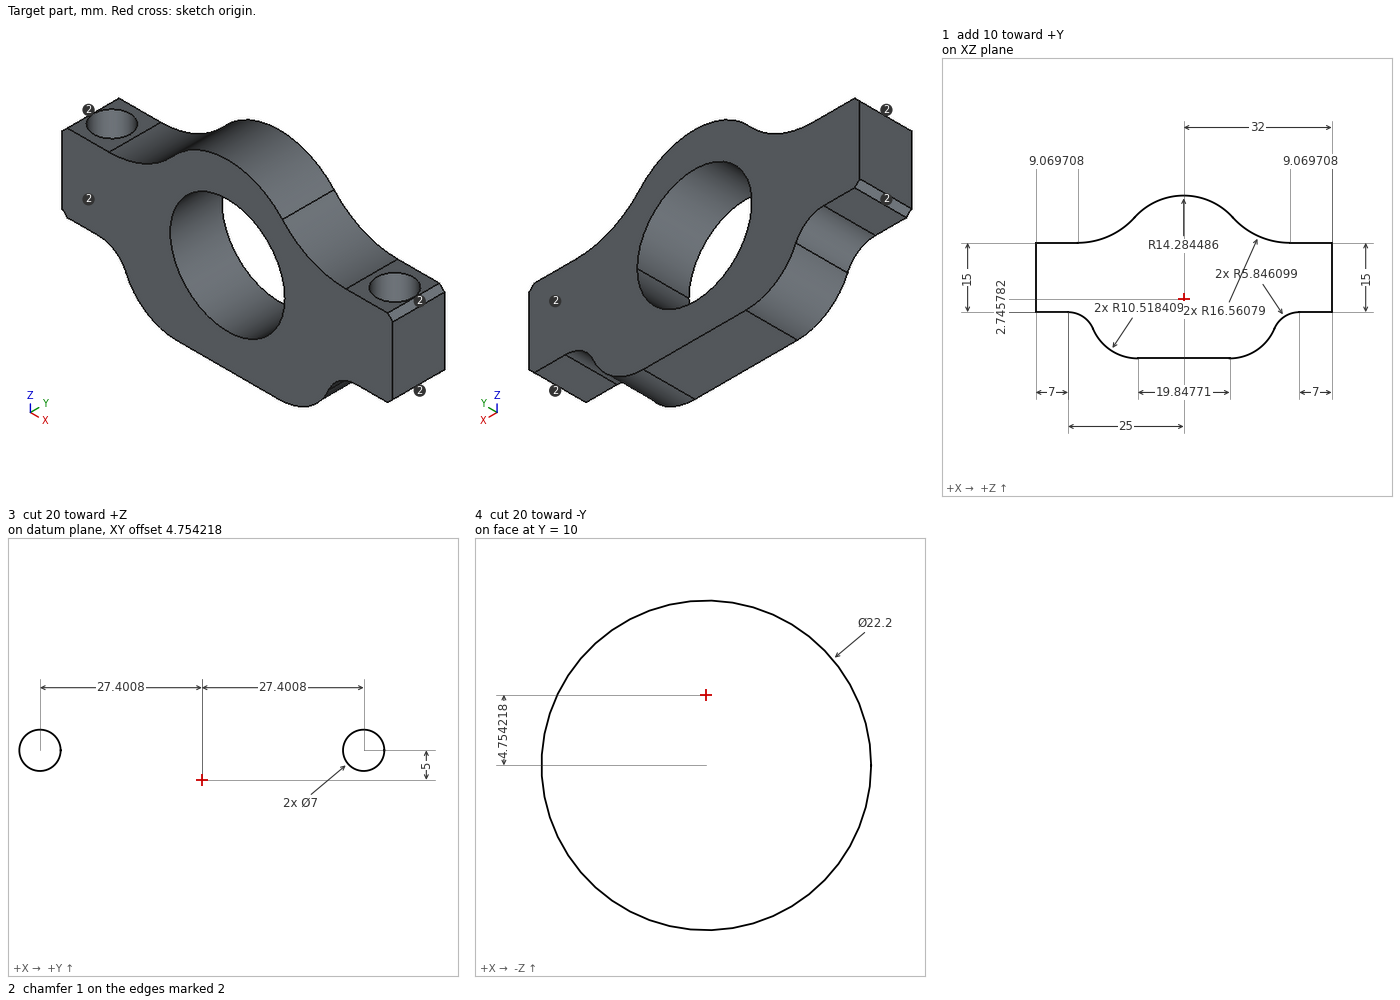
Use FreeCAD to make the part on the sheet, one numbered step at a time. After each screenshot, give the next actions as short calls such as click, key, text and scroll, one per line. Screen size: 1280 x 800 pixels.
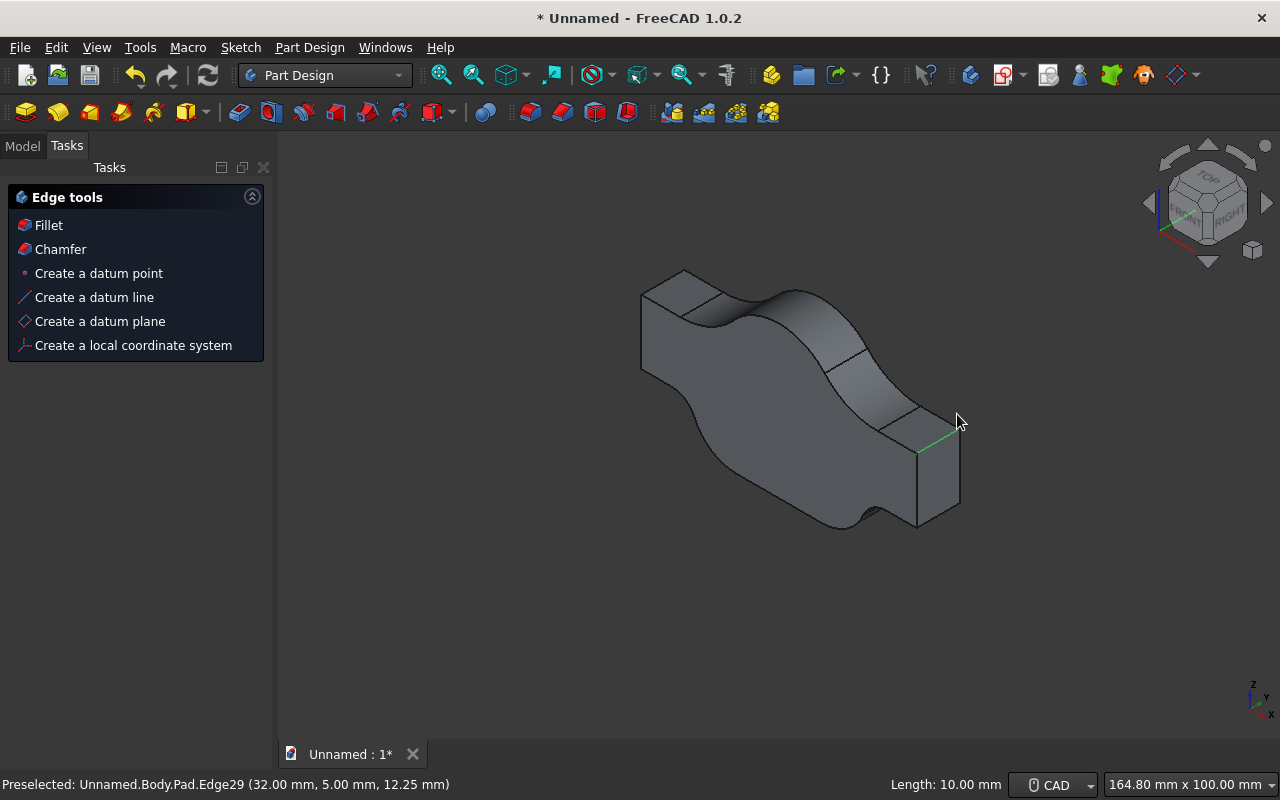
key(2)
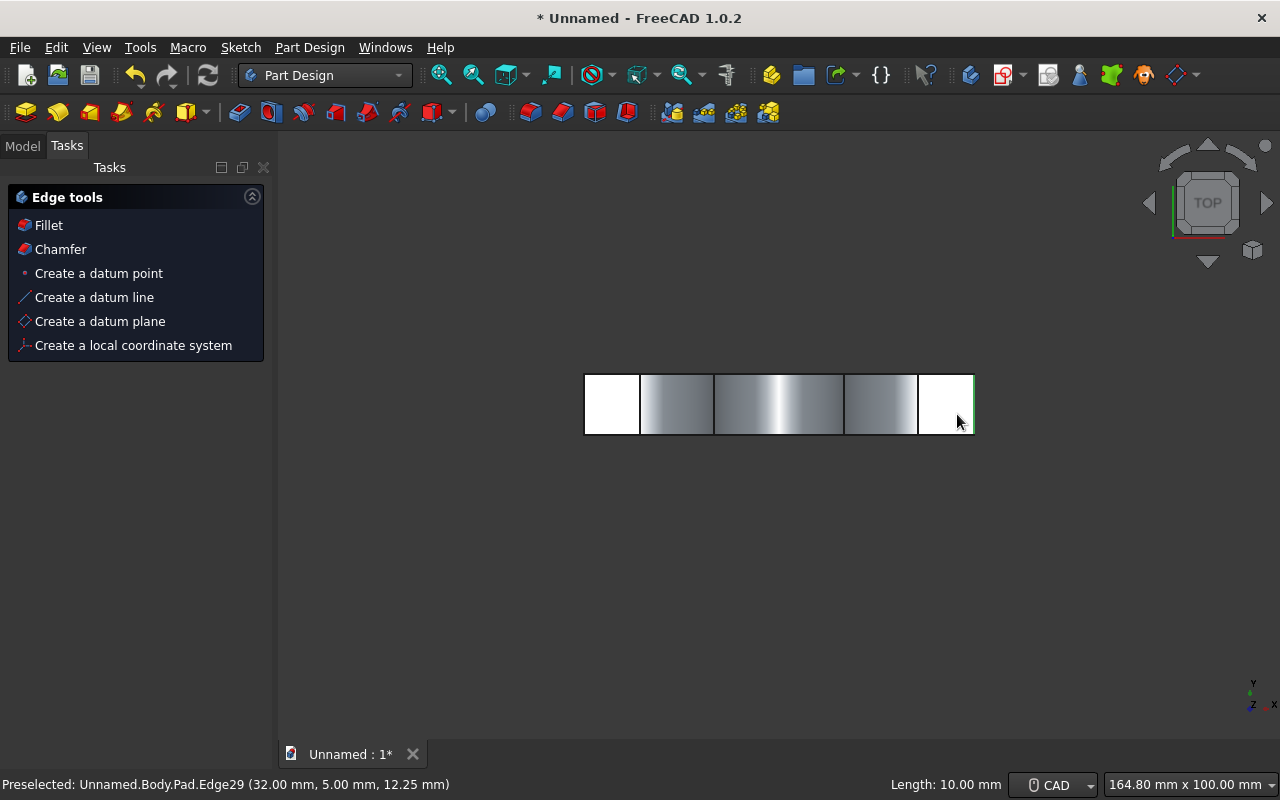
click(442, 76)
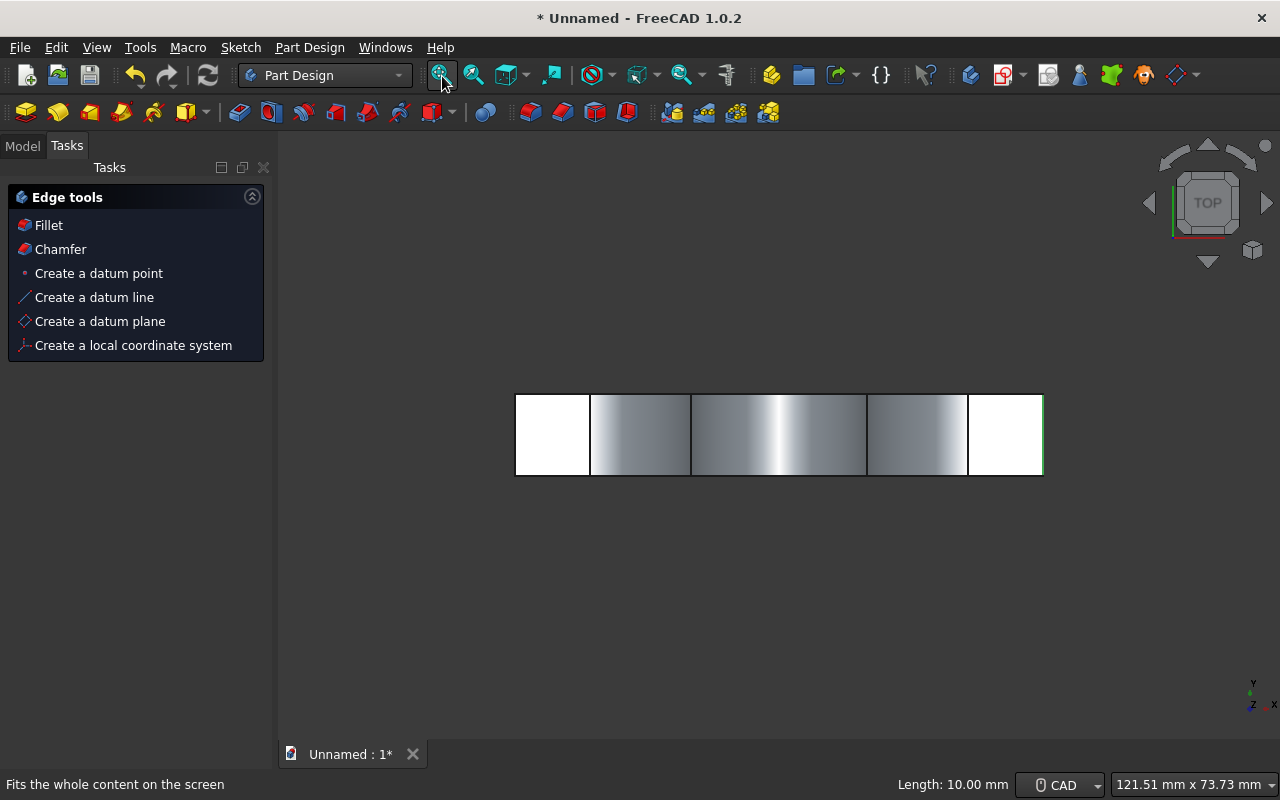
click(515, 434, ctrl)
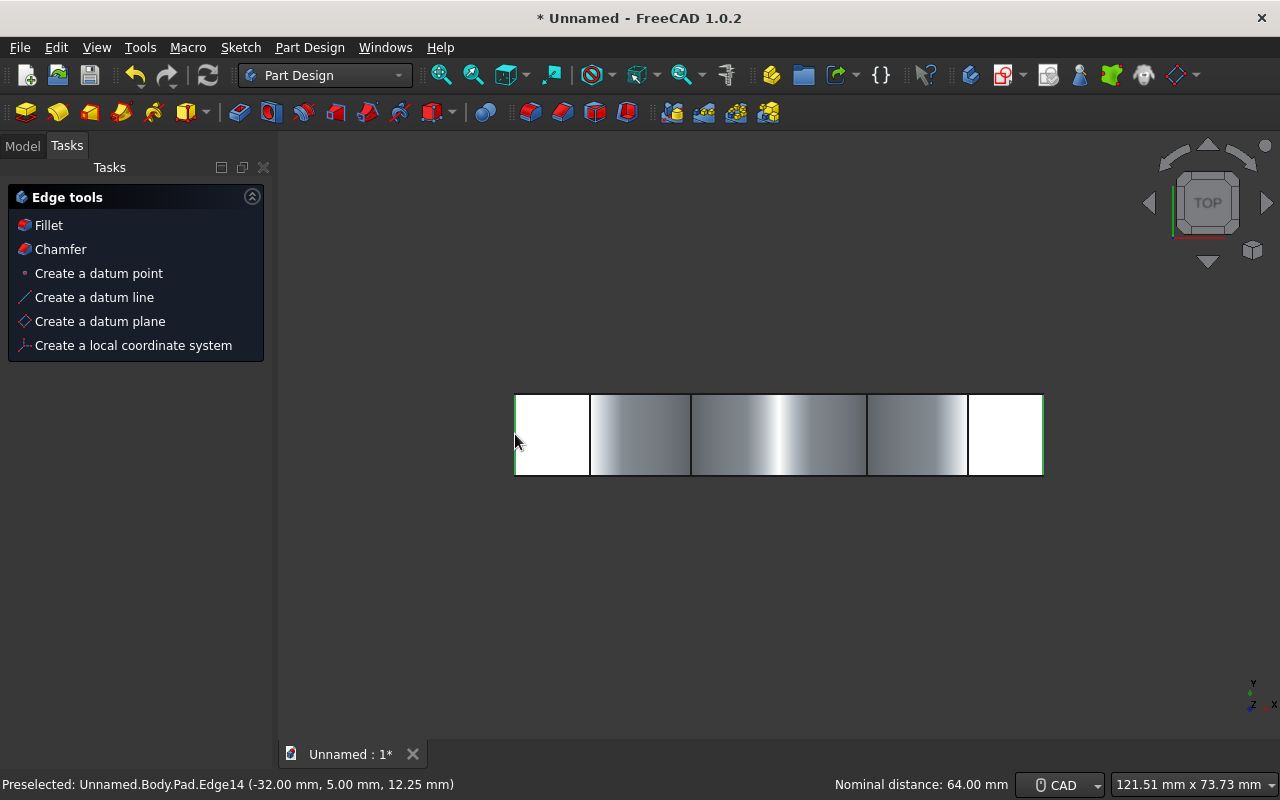
key(1)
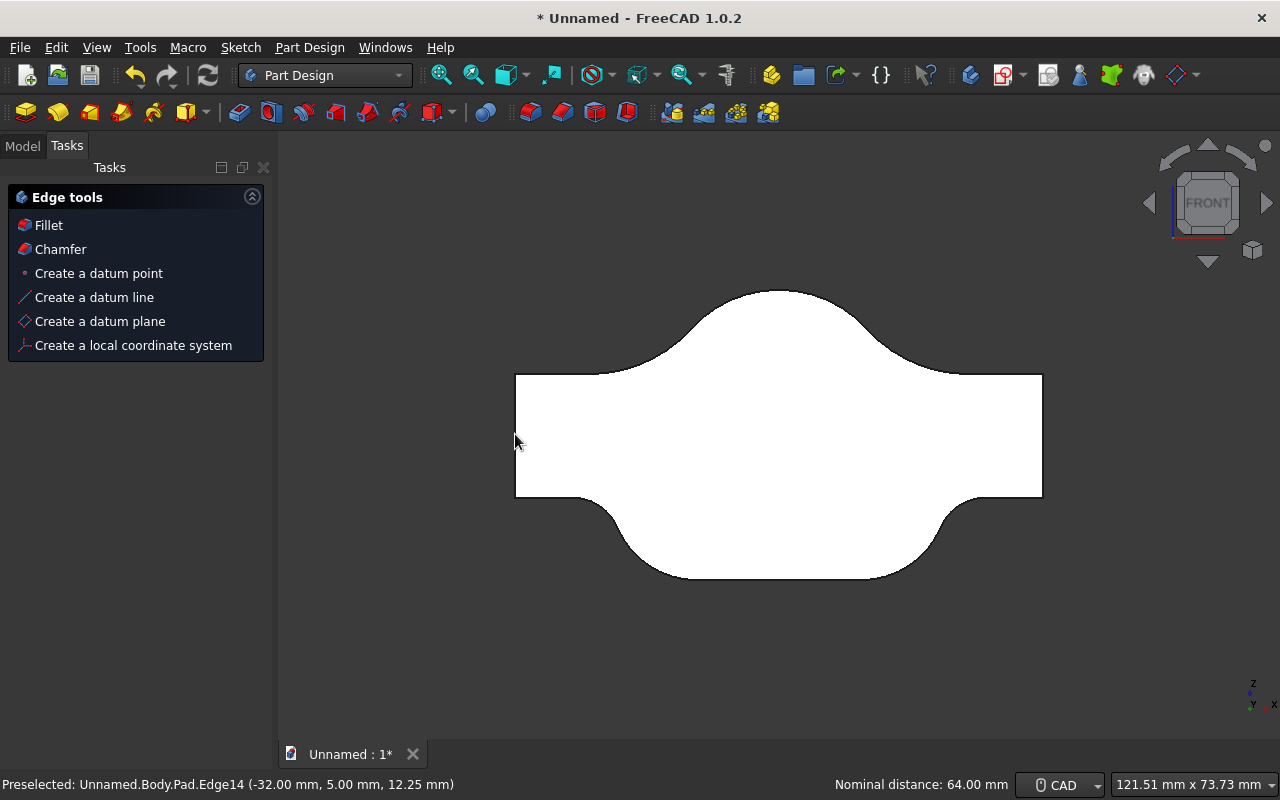
key(3)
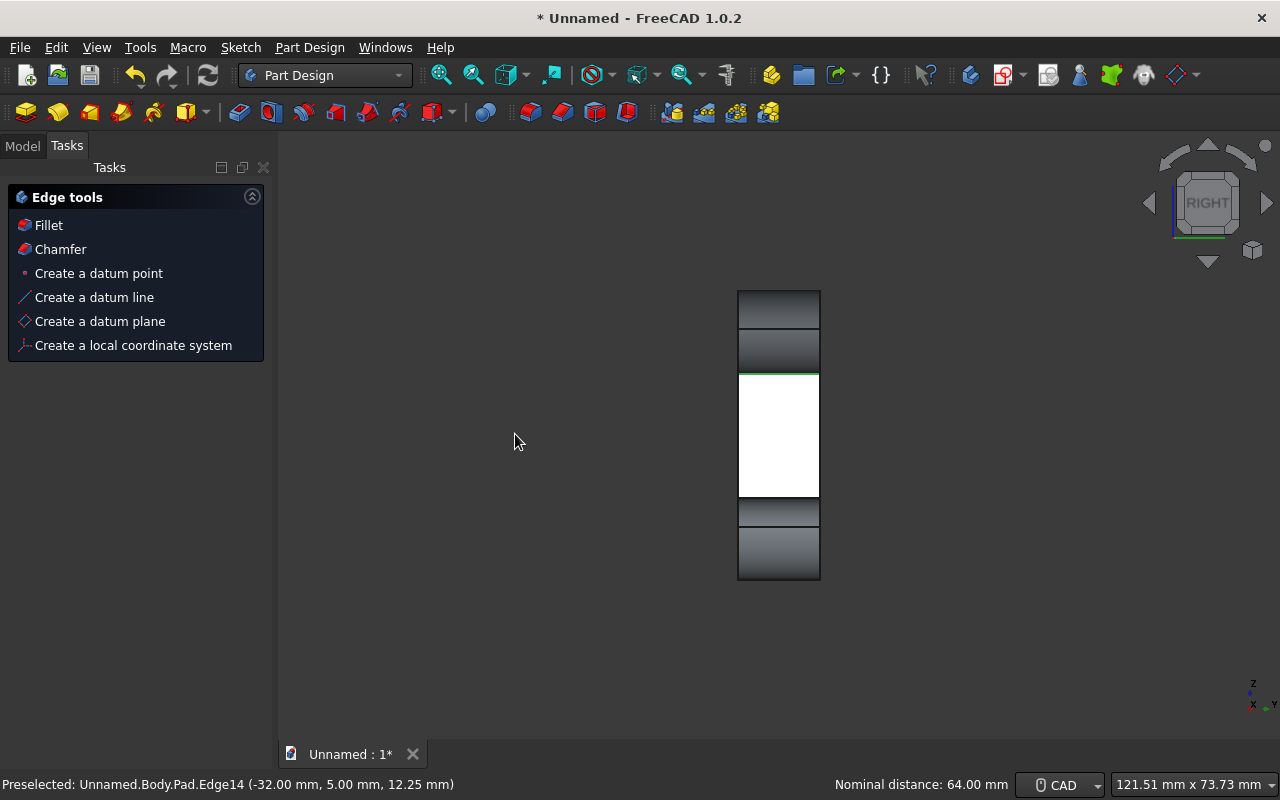
click(779, 497, ctrl)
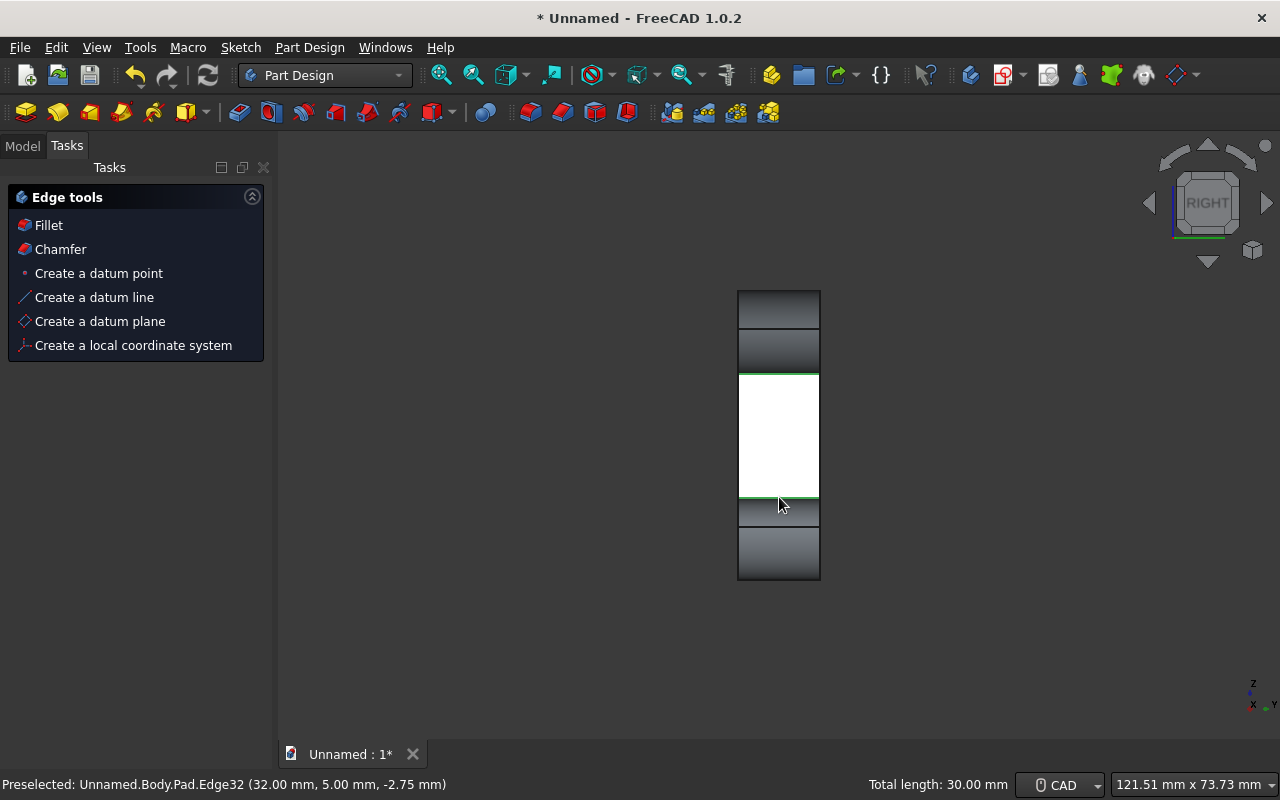
key(5)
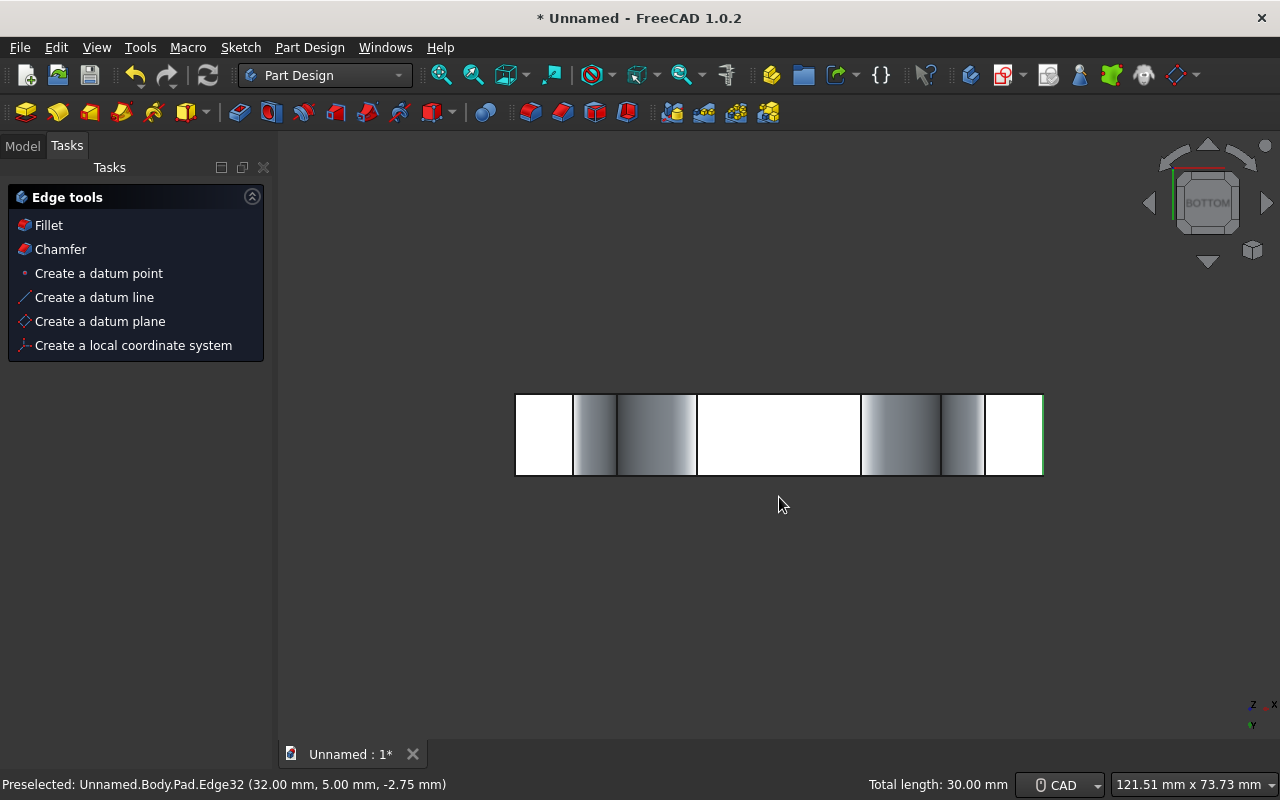
click(515, 434, ctrl)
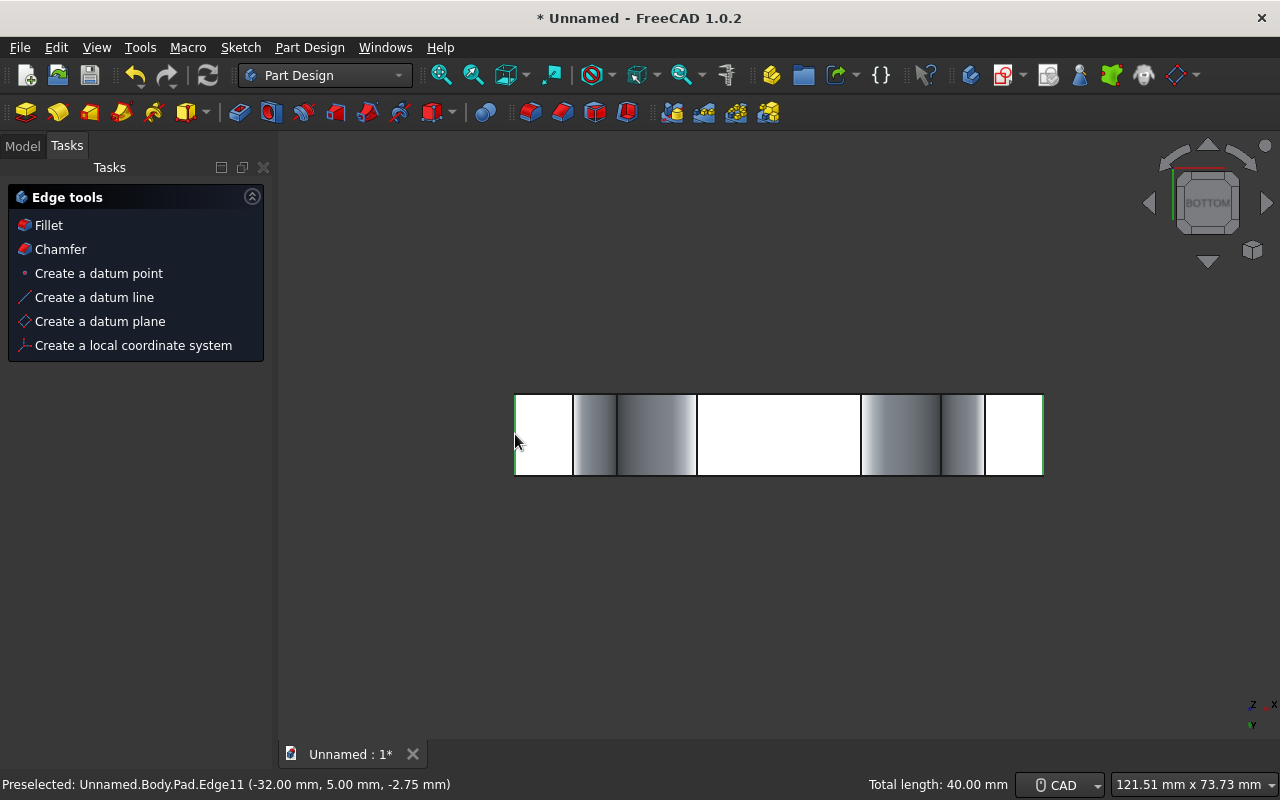
click(564, 112)